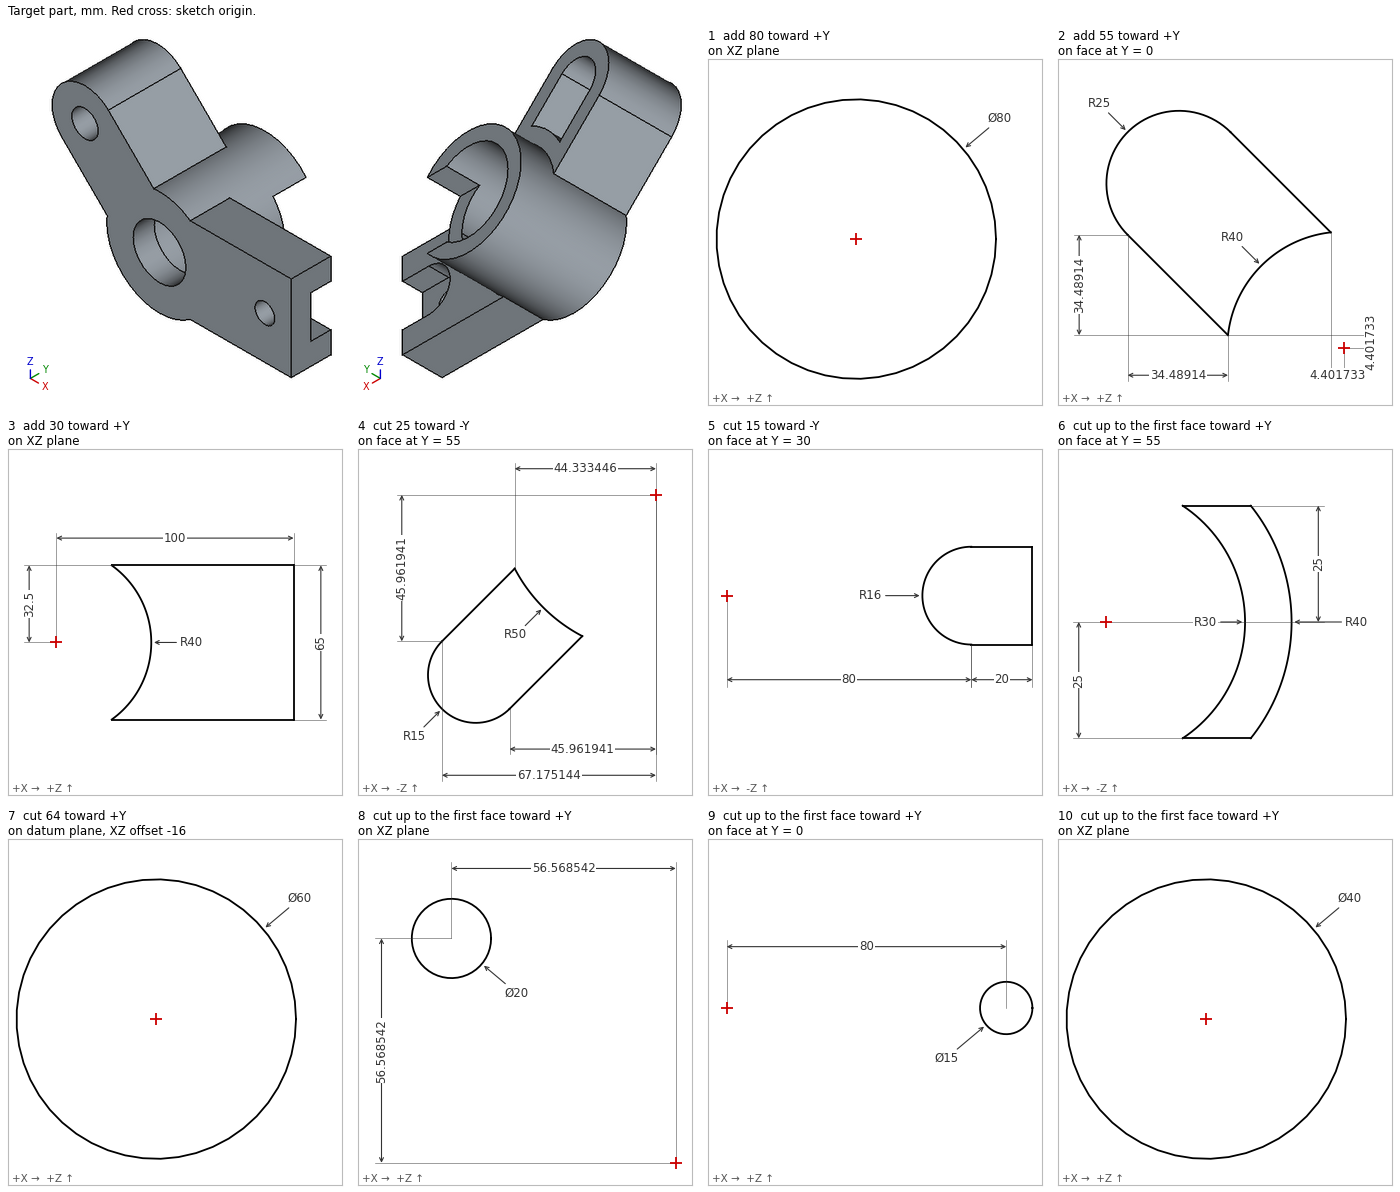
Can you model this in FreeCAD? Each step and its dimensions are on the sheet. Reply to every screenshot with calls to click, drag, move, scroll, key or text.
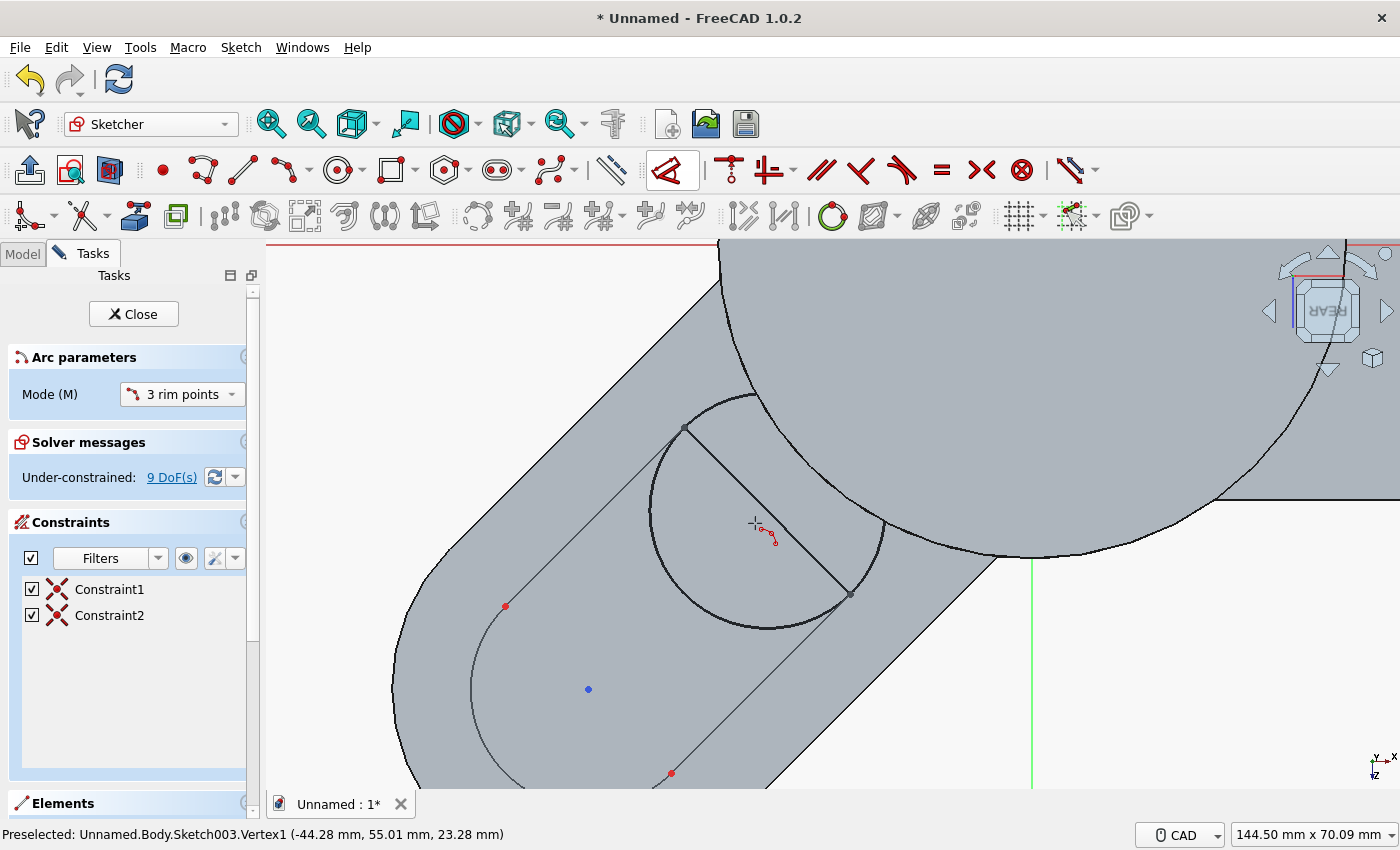
click(755, 522)
key(Escape)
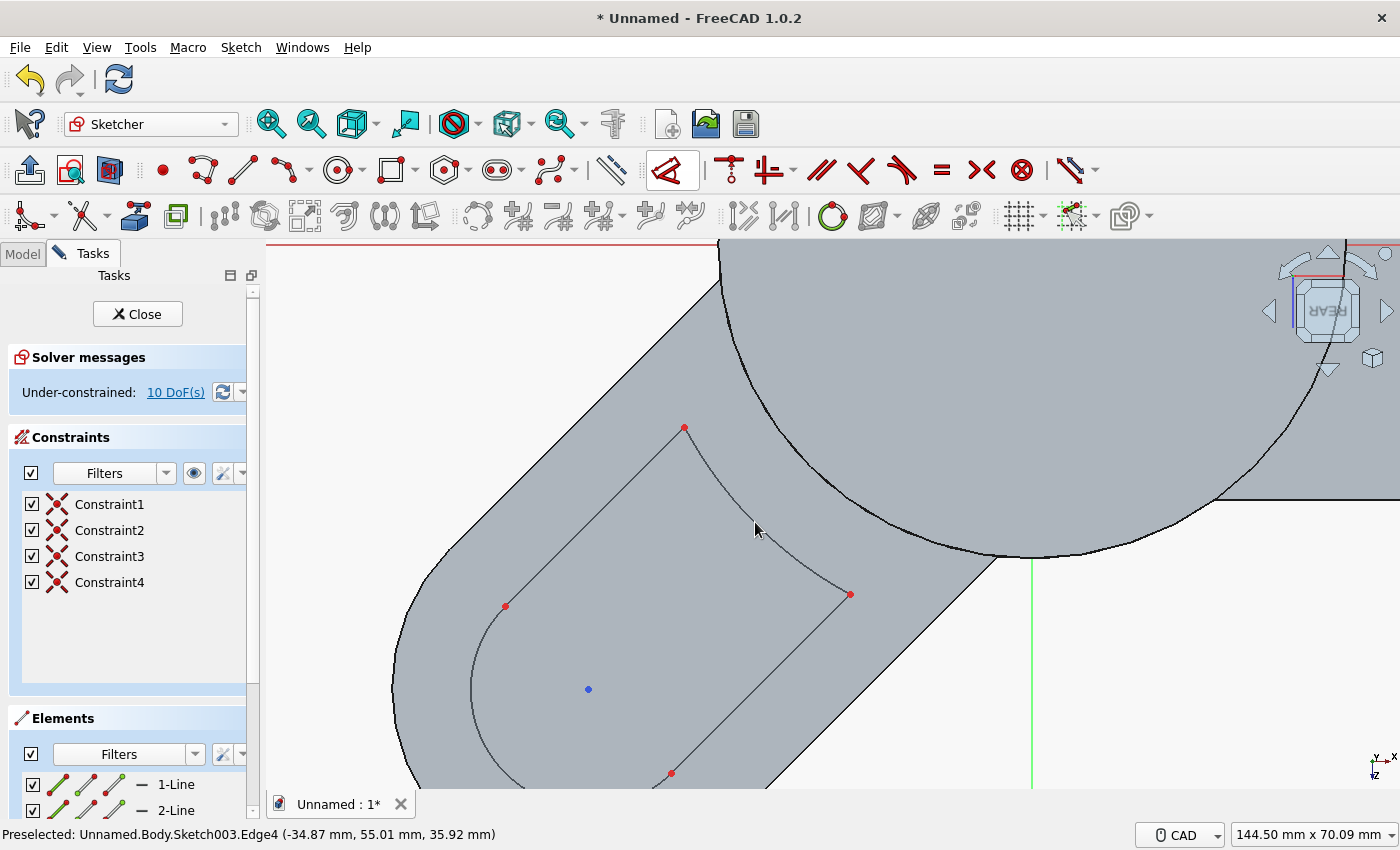
click(631, 481)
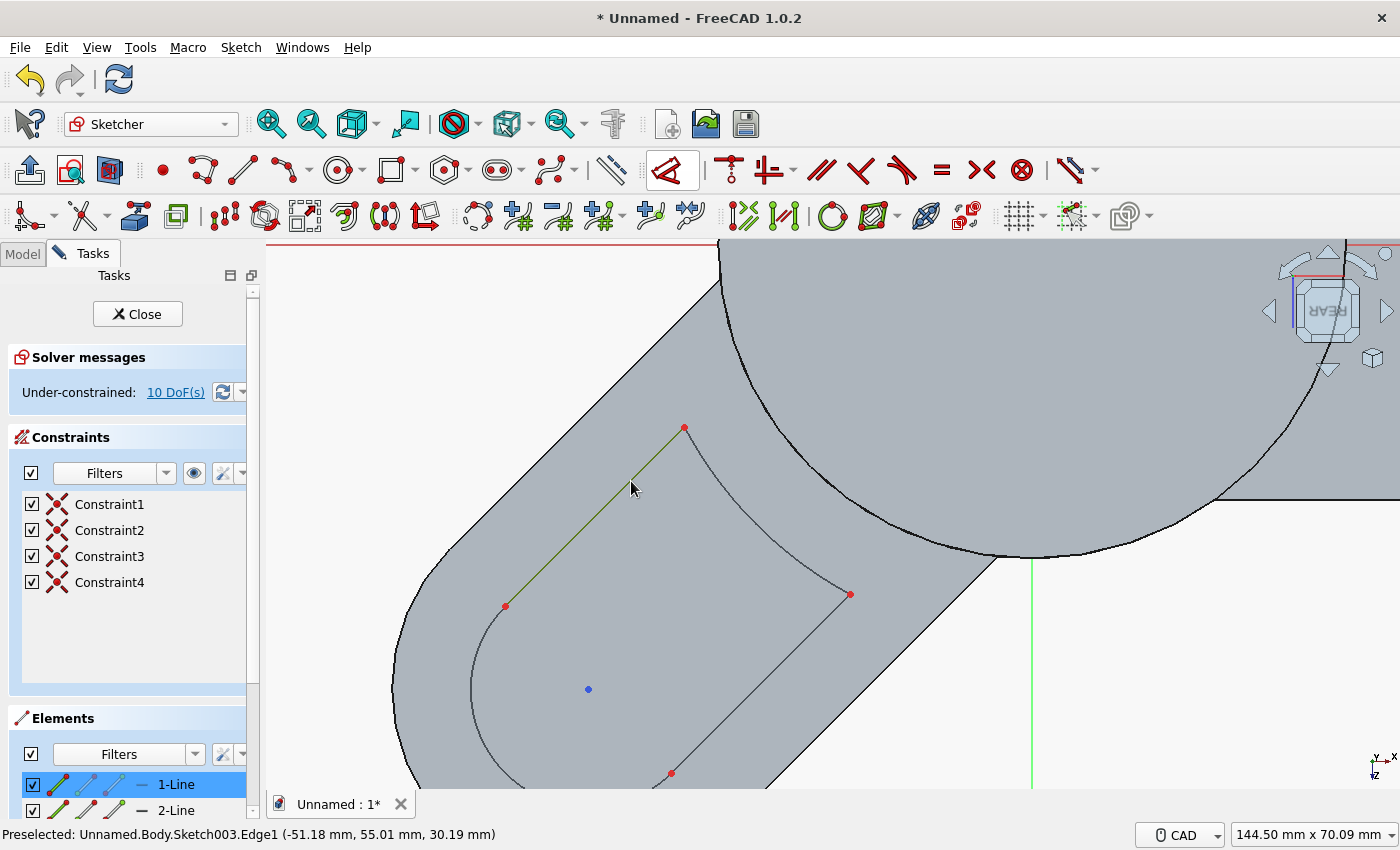
click(472, 708)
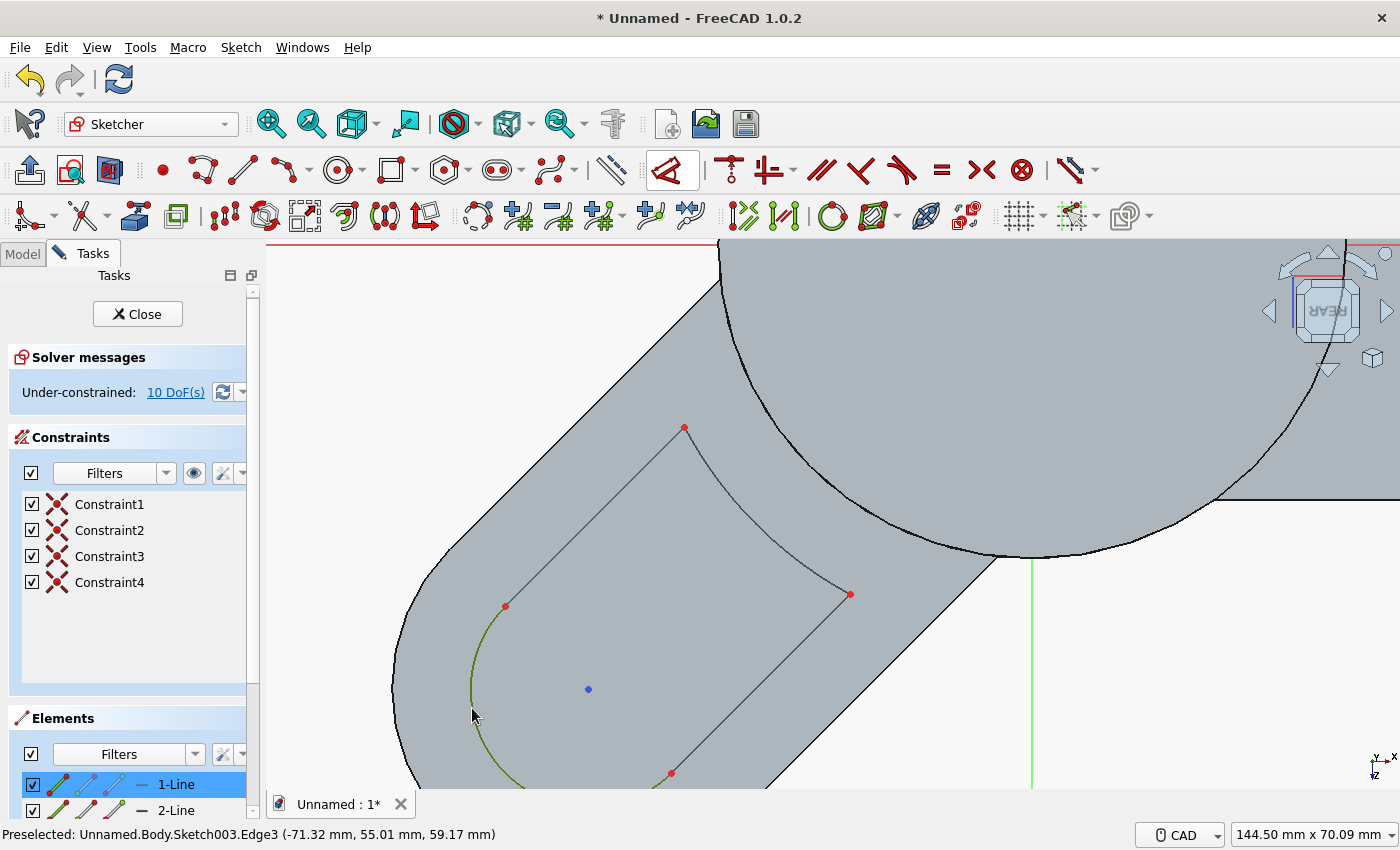
click(902, 170)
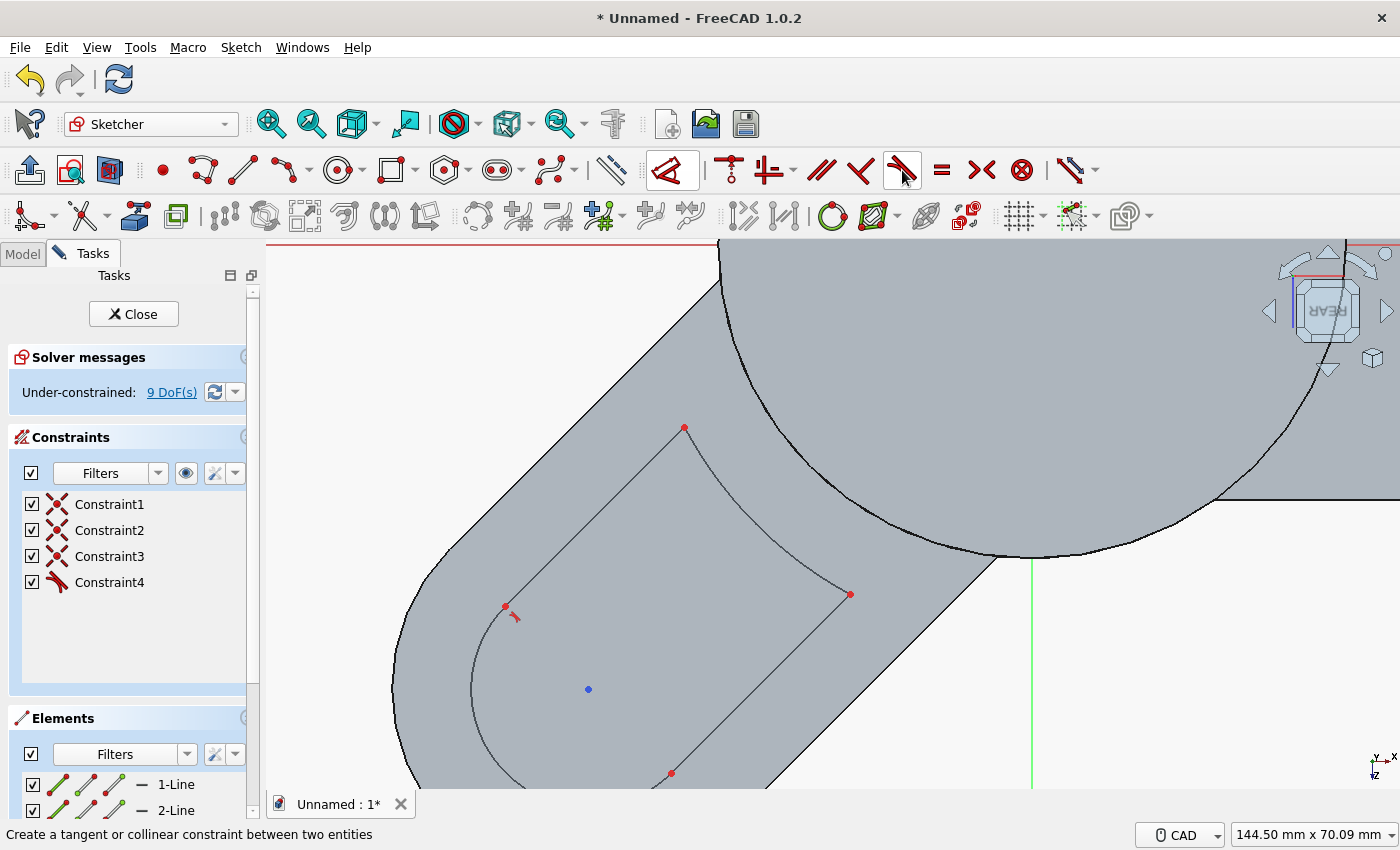
click(725, 720)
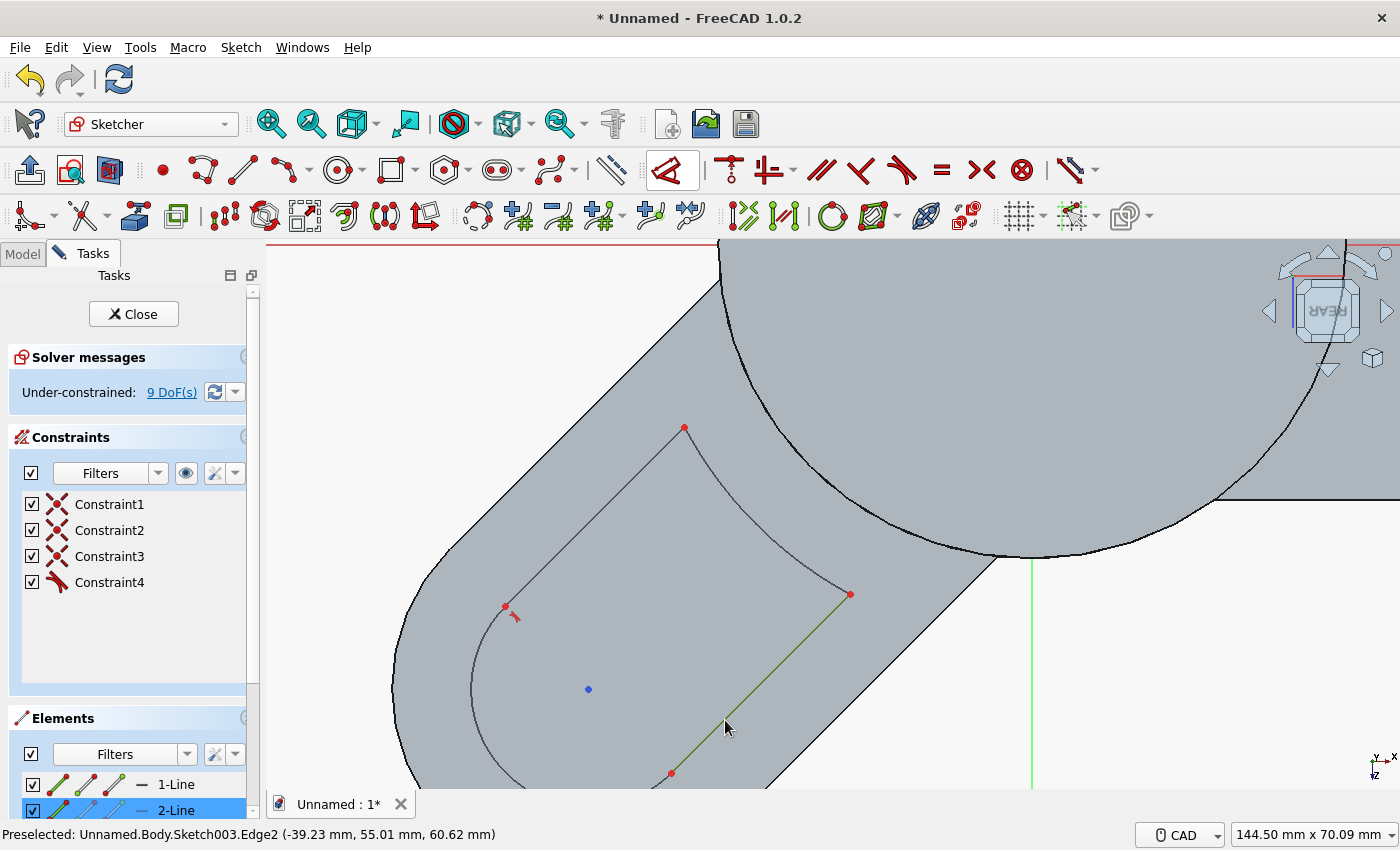
click(473, 708)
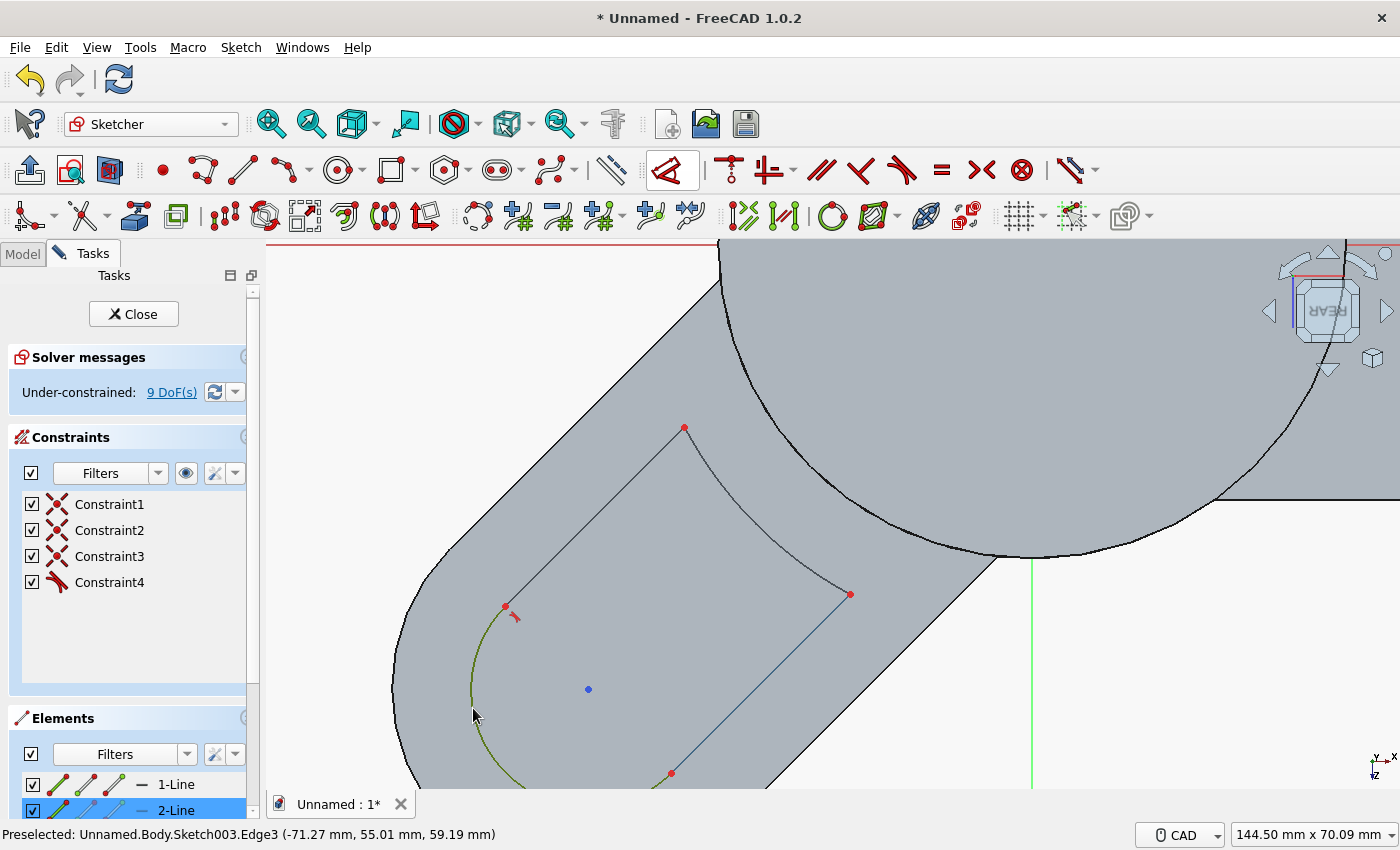
key(t)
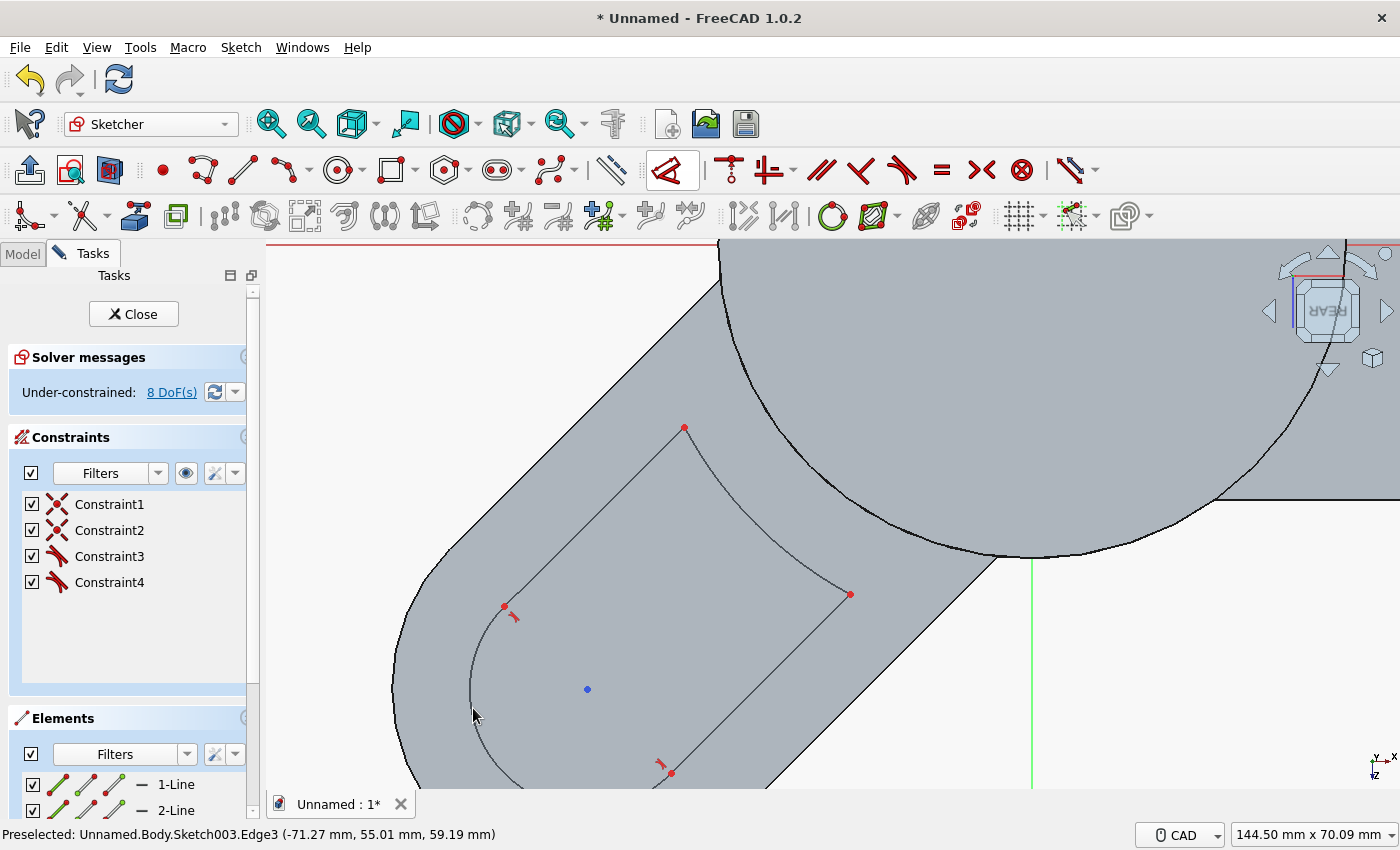
scroll(756, 526, down, 2)